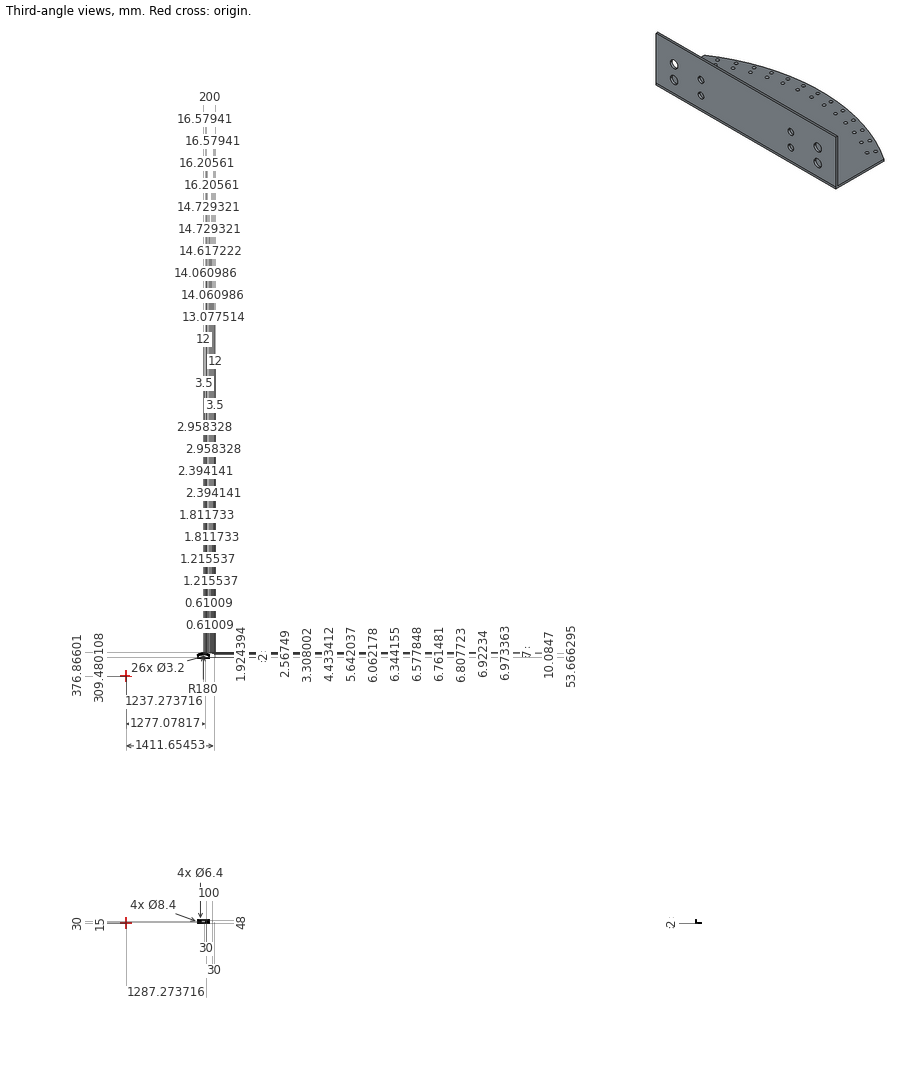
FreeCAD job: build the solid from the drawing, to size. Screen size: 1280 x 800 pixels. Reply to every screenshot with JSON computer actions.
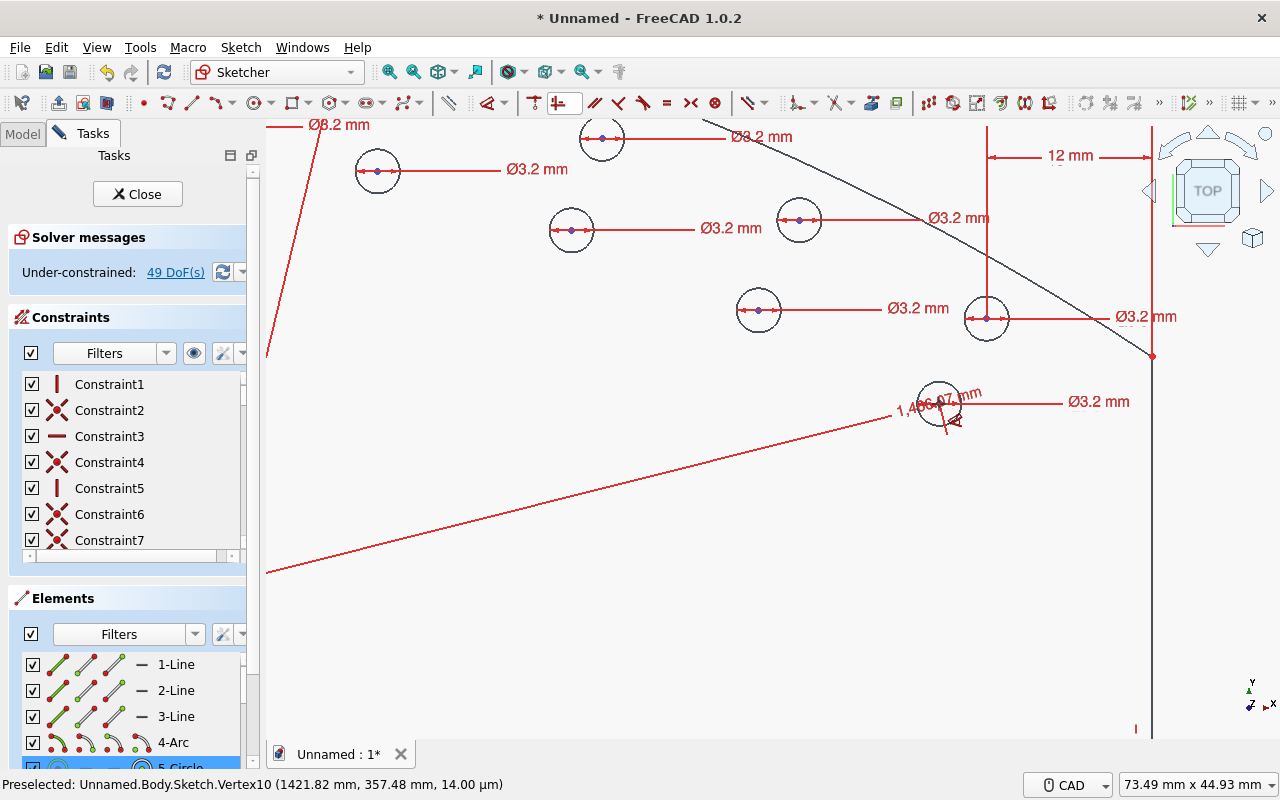
{"action": "left_click", "coordinate": [987, 319]}
{"action": "left_click", "coordinate": [963, 285]}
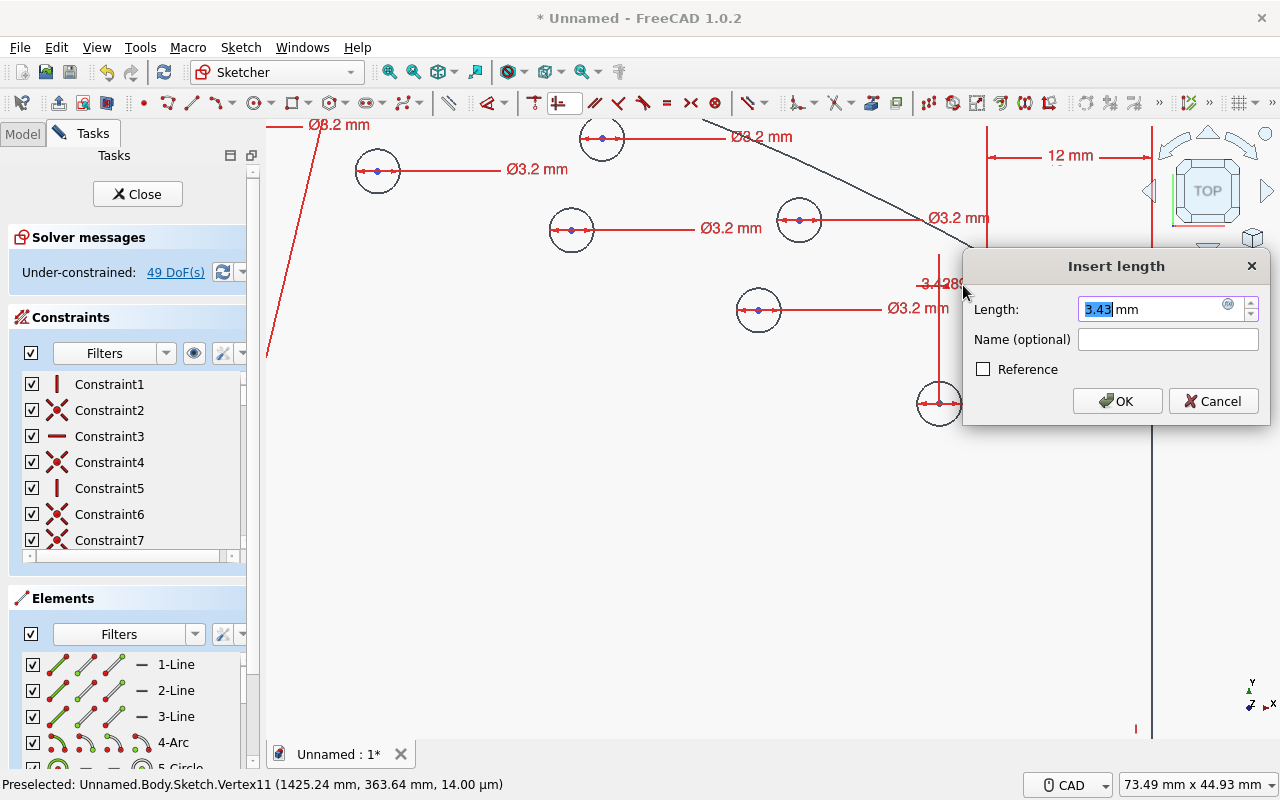
{"action": "type", "text": "3.5"}
{"action": "key", "text": "Return"}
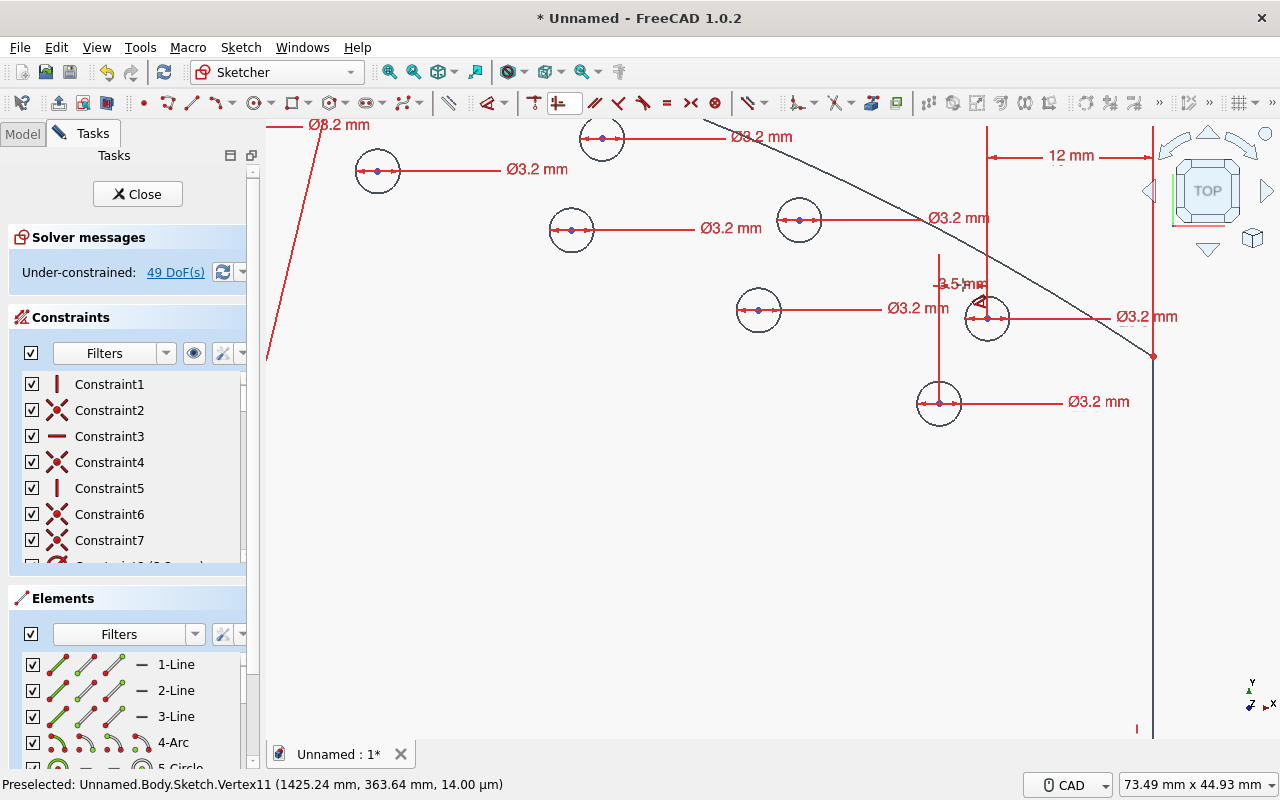
{"action": "scroll", "coordinate": [940, 407], "scroll_direction": "down", "scroll_amount": 8}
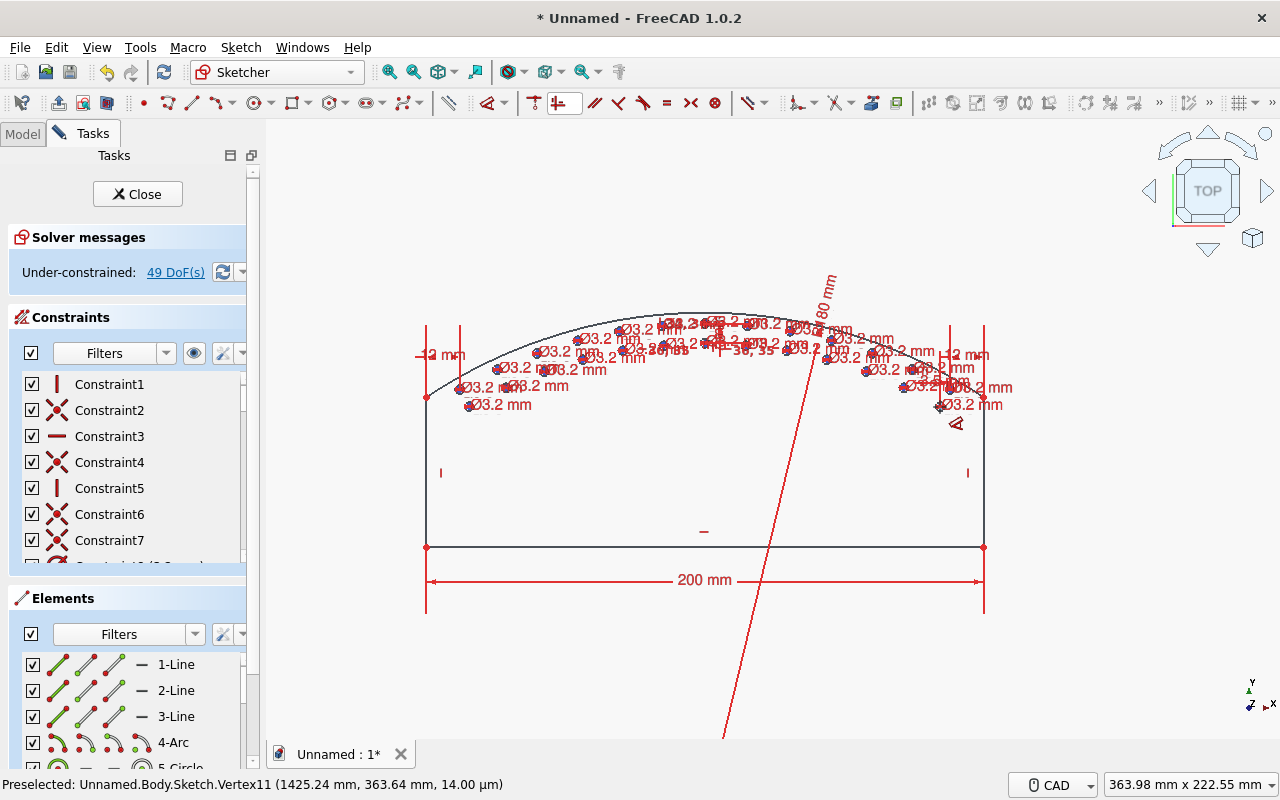
{"action": "scroll", "coordinate": [469, 407], "scroll_direction": "up", "scroll_amount": 8}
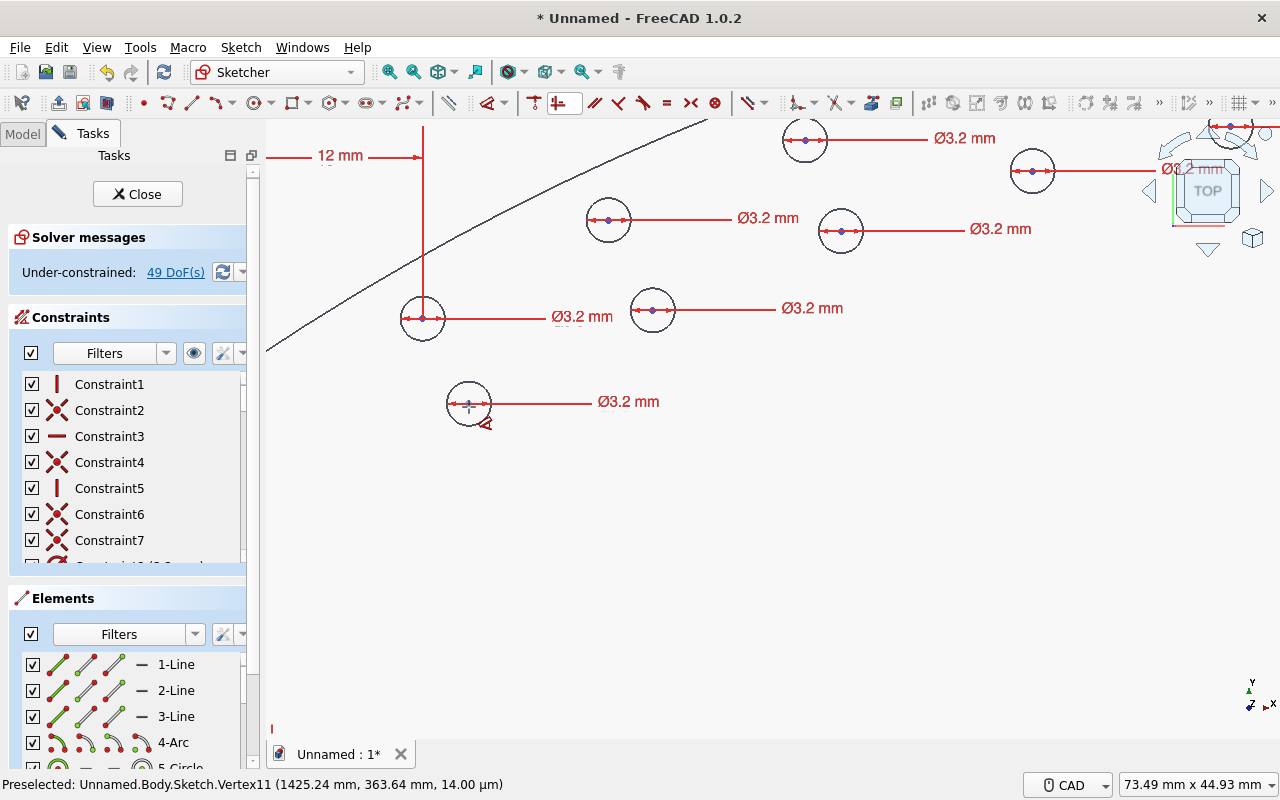
{"action": "left_click", "coordinate": [469, 404]}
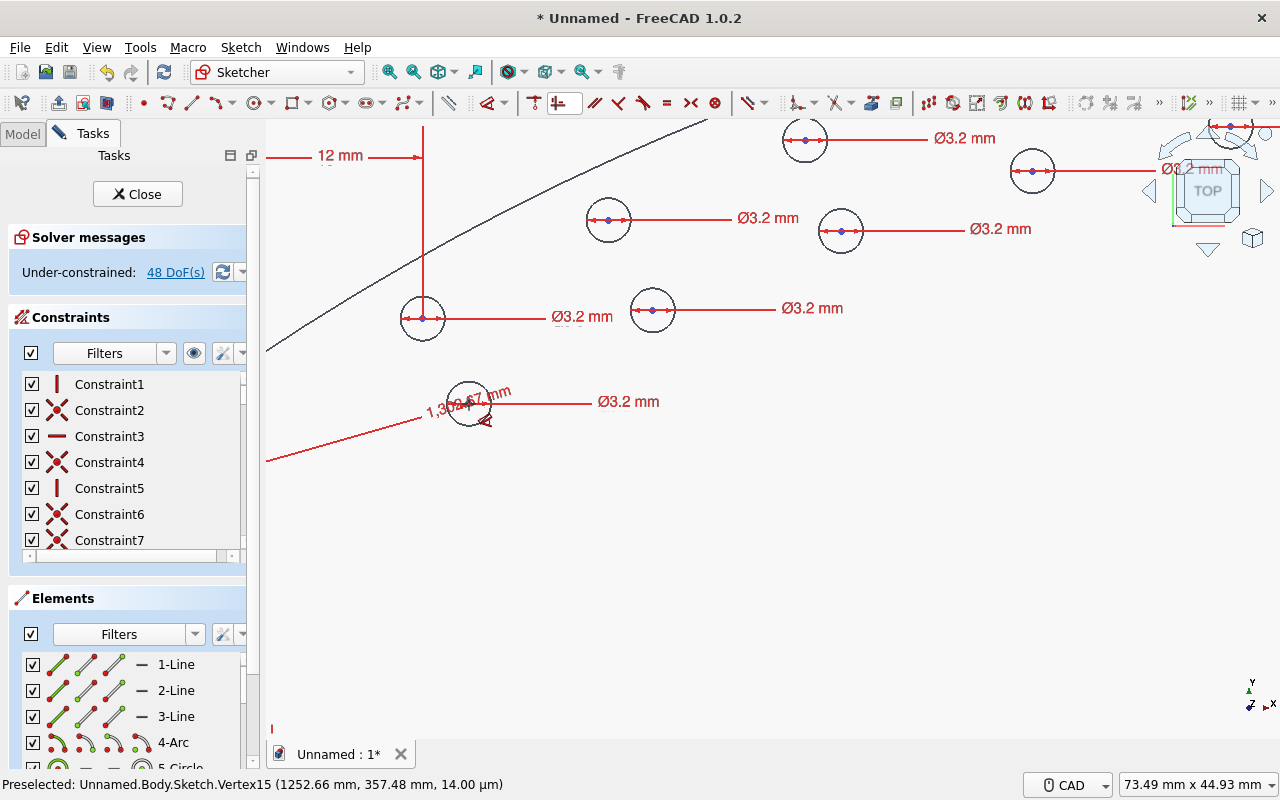
{"action": "left_click", "coordinate": [423, 319]}
{"action": "left_click", "coordinate": [446, 285]}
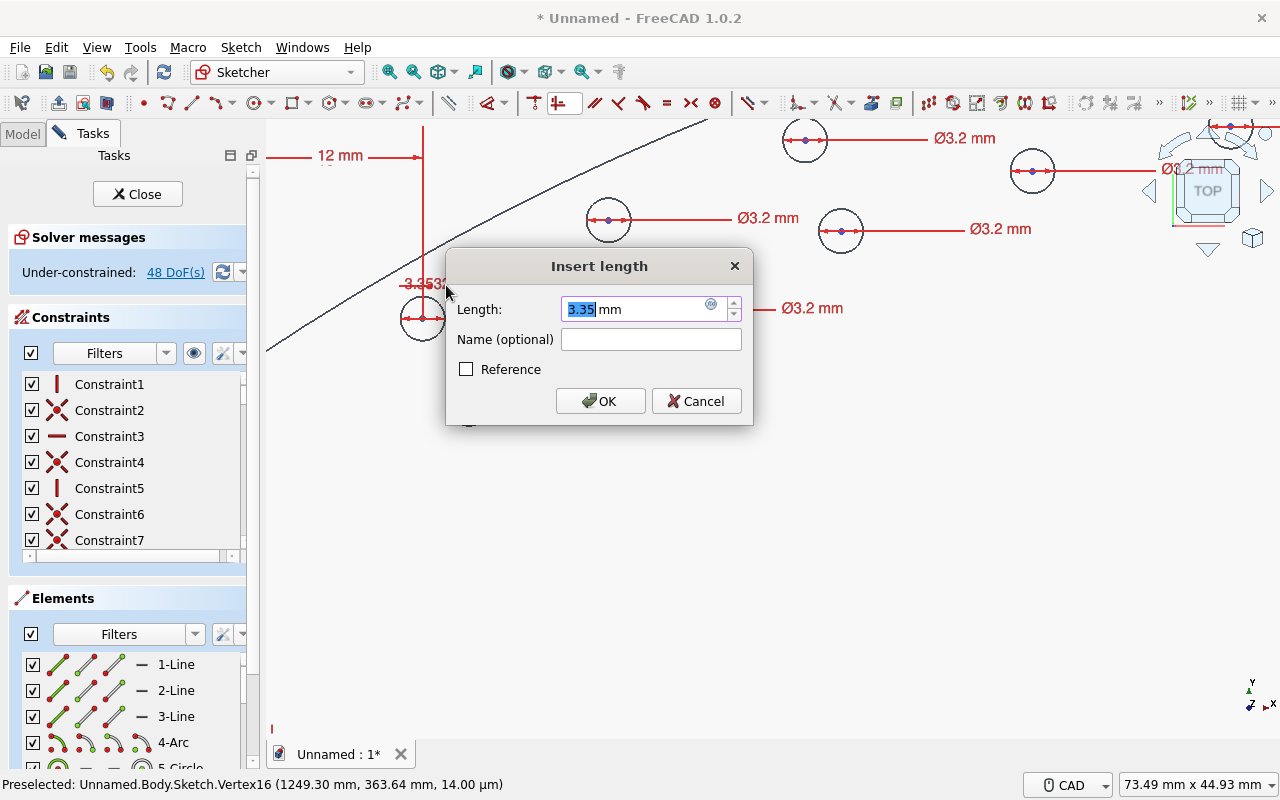
{"action": "type", "text": "3.5"}
{"action": "key", "text": "Return"}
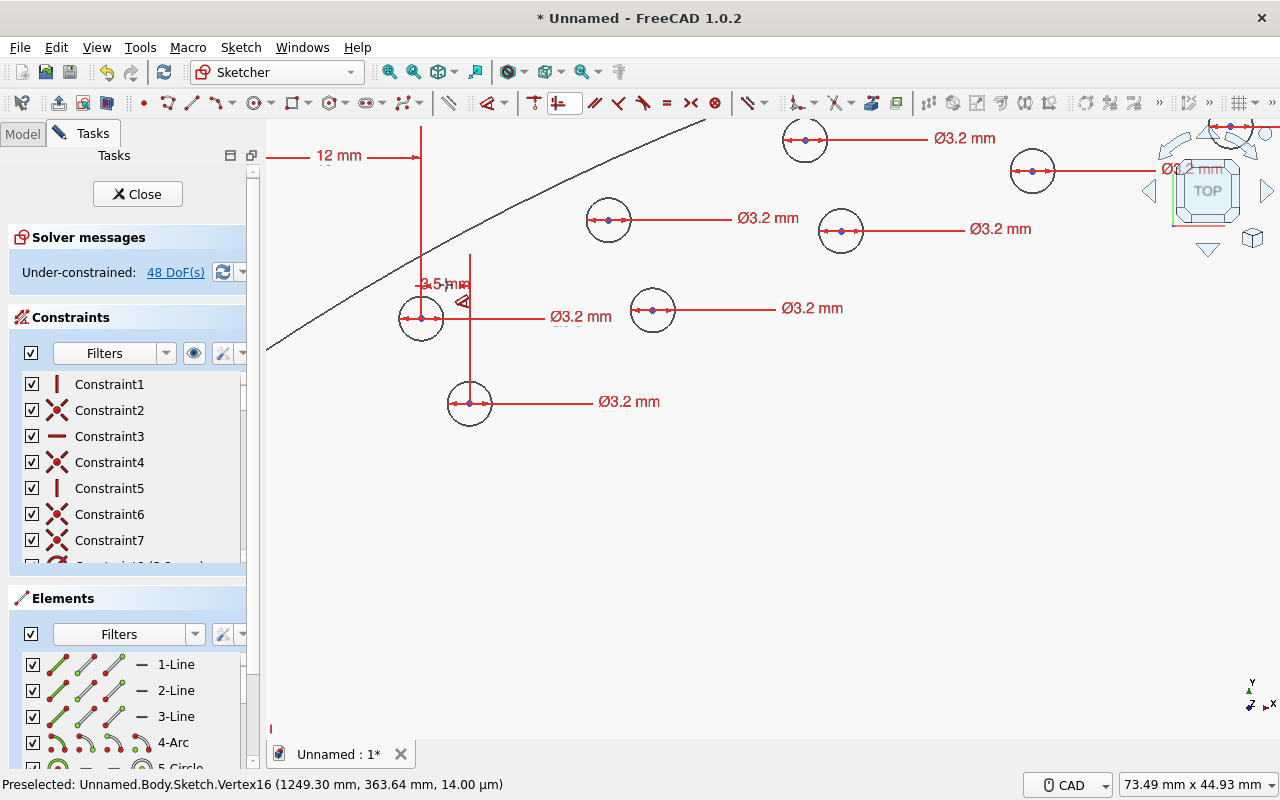
{"action": "scroll", "coordinate": [469, 407], "scroll_direction": "down", "scroll_amount": 8}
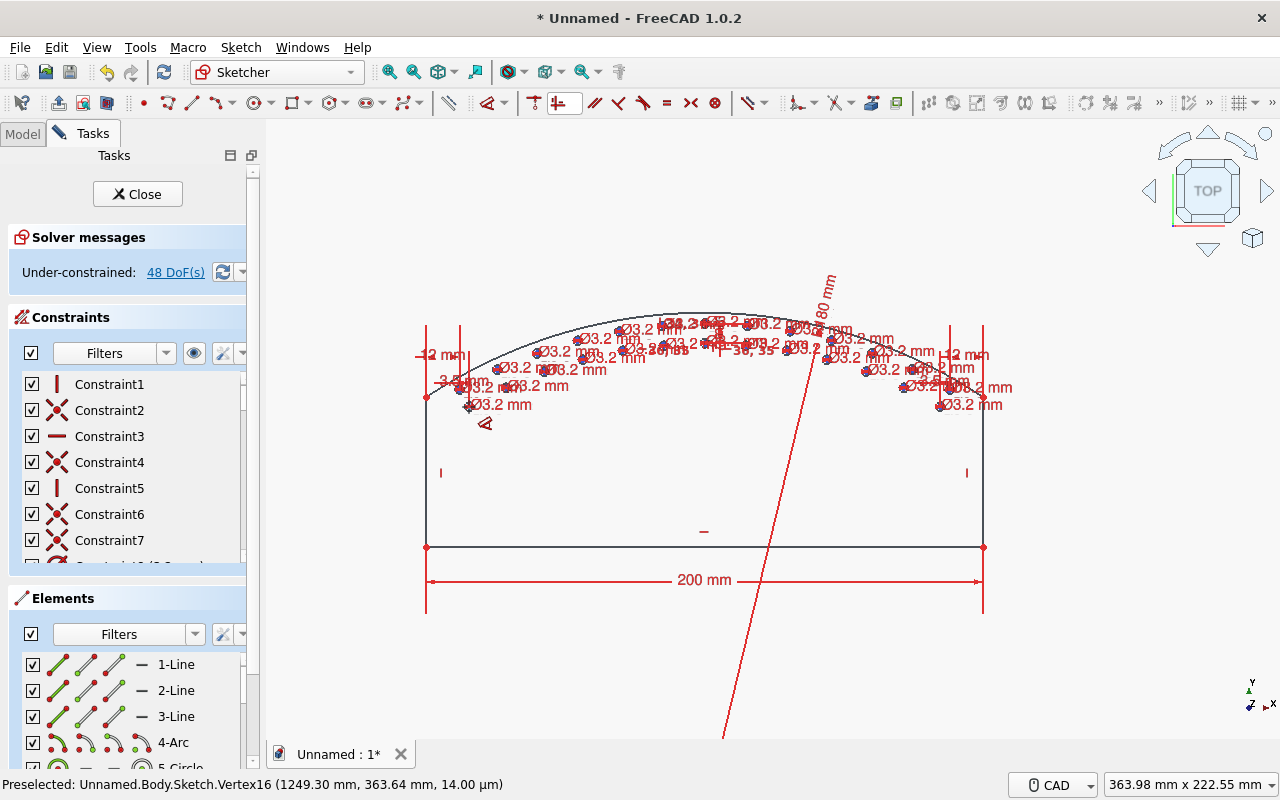
{"action": "scroll", "coordinate": [912, 370], "scroll_direction": "up", "scroll_amount": 4}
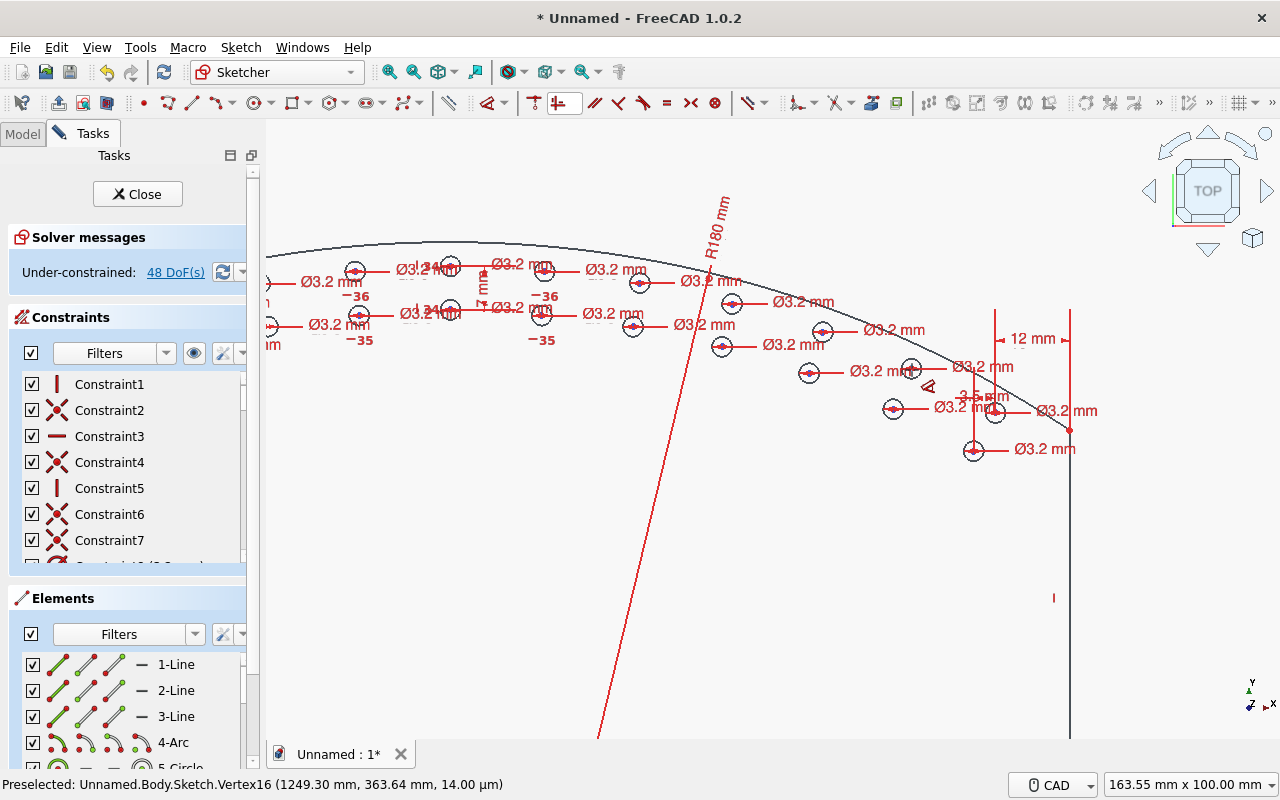
{"action": "left_click", "coordinate": [912, 369]}